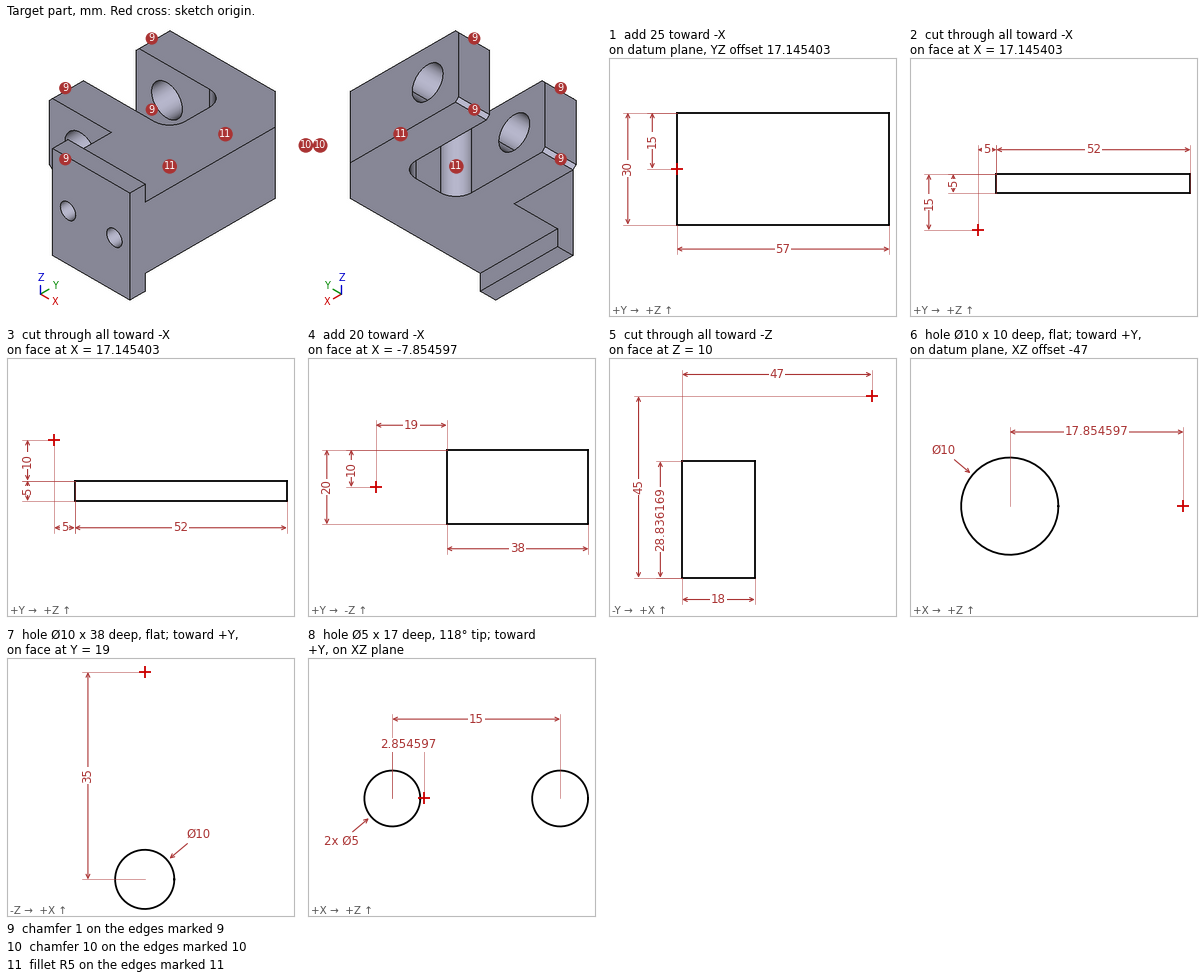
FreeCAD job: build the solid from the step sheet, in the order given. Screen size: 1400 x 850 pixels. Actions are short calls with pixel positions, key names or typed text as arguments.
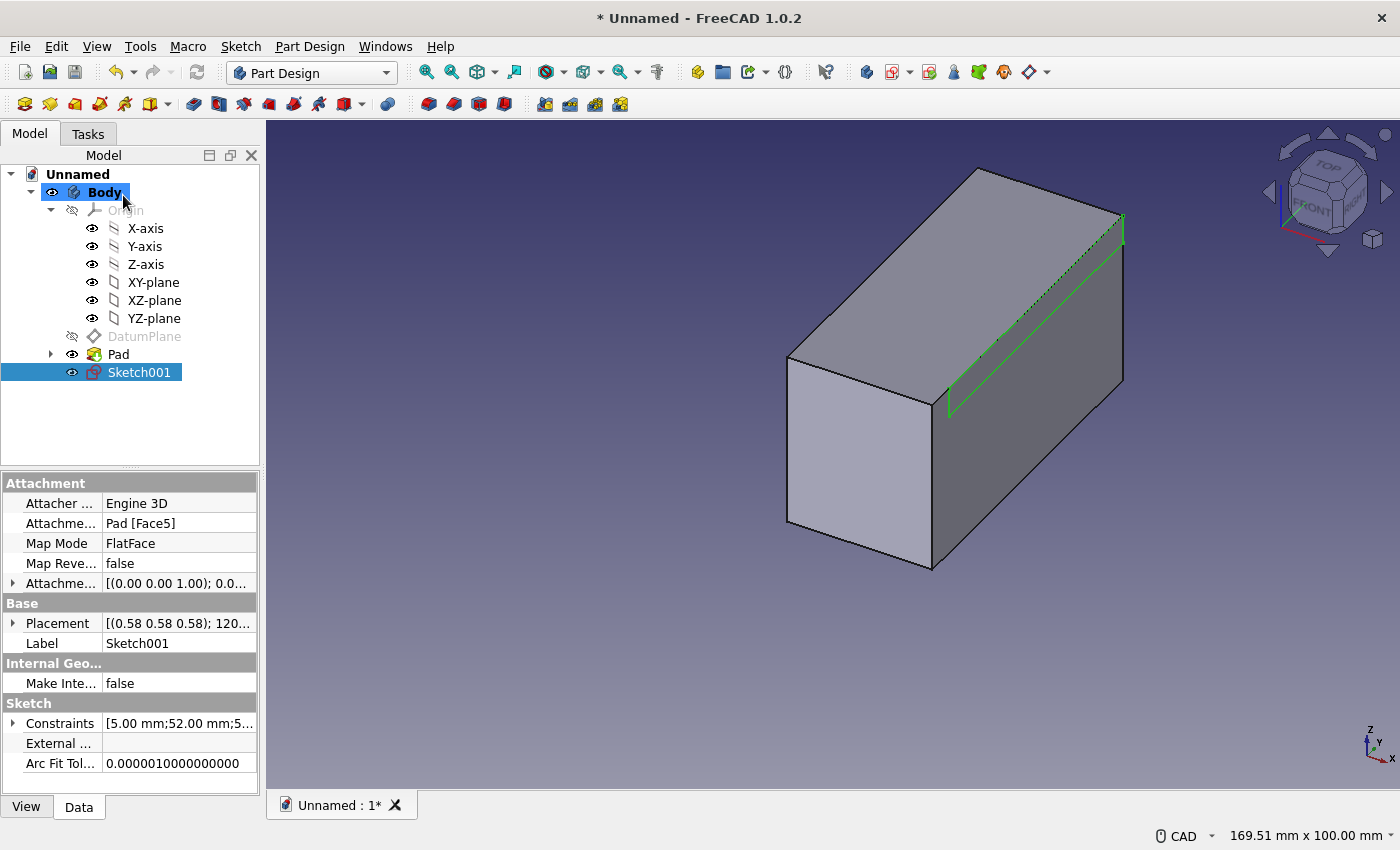
click(194, 104)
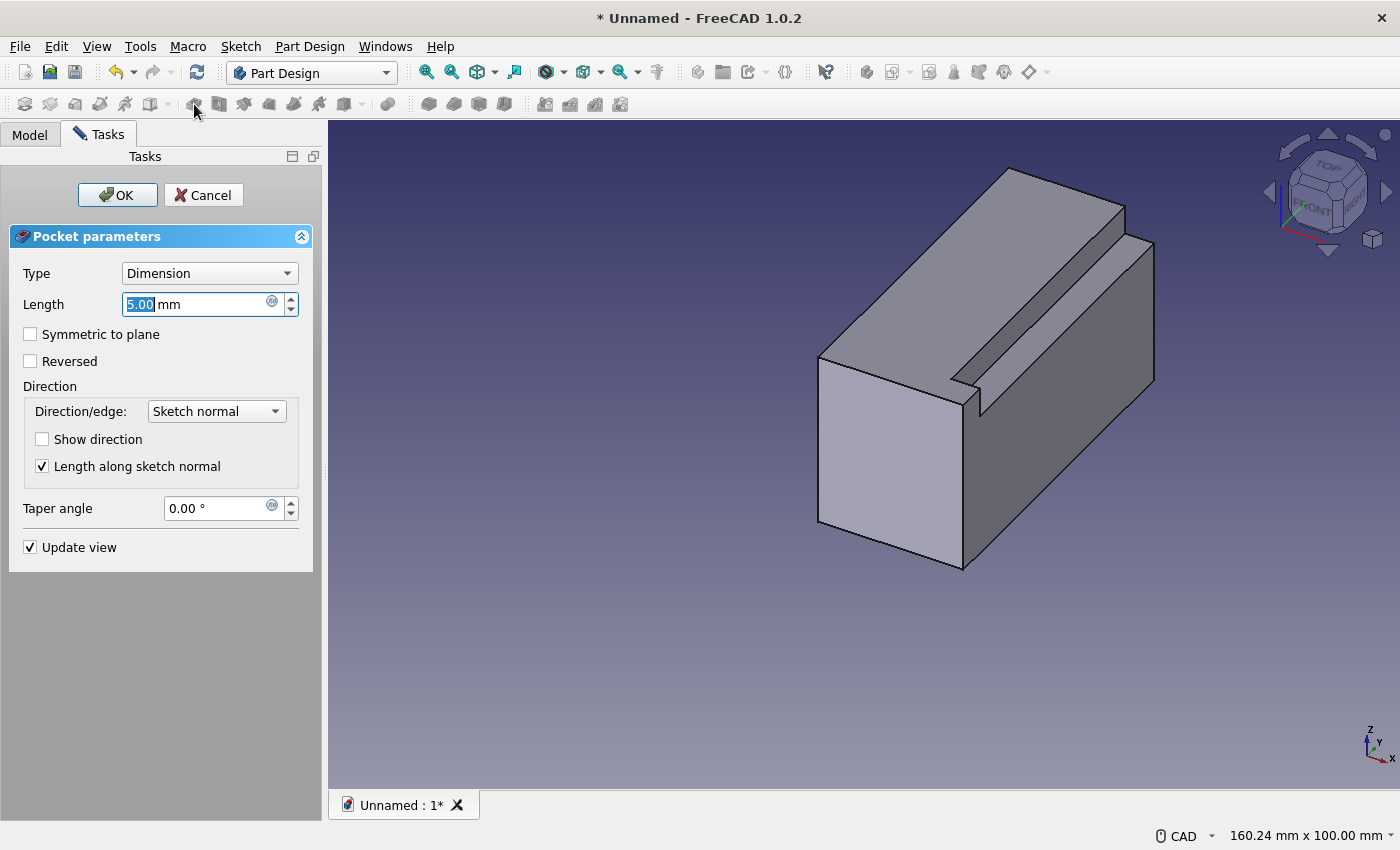
click(210, 274)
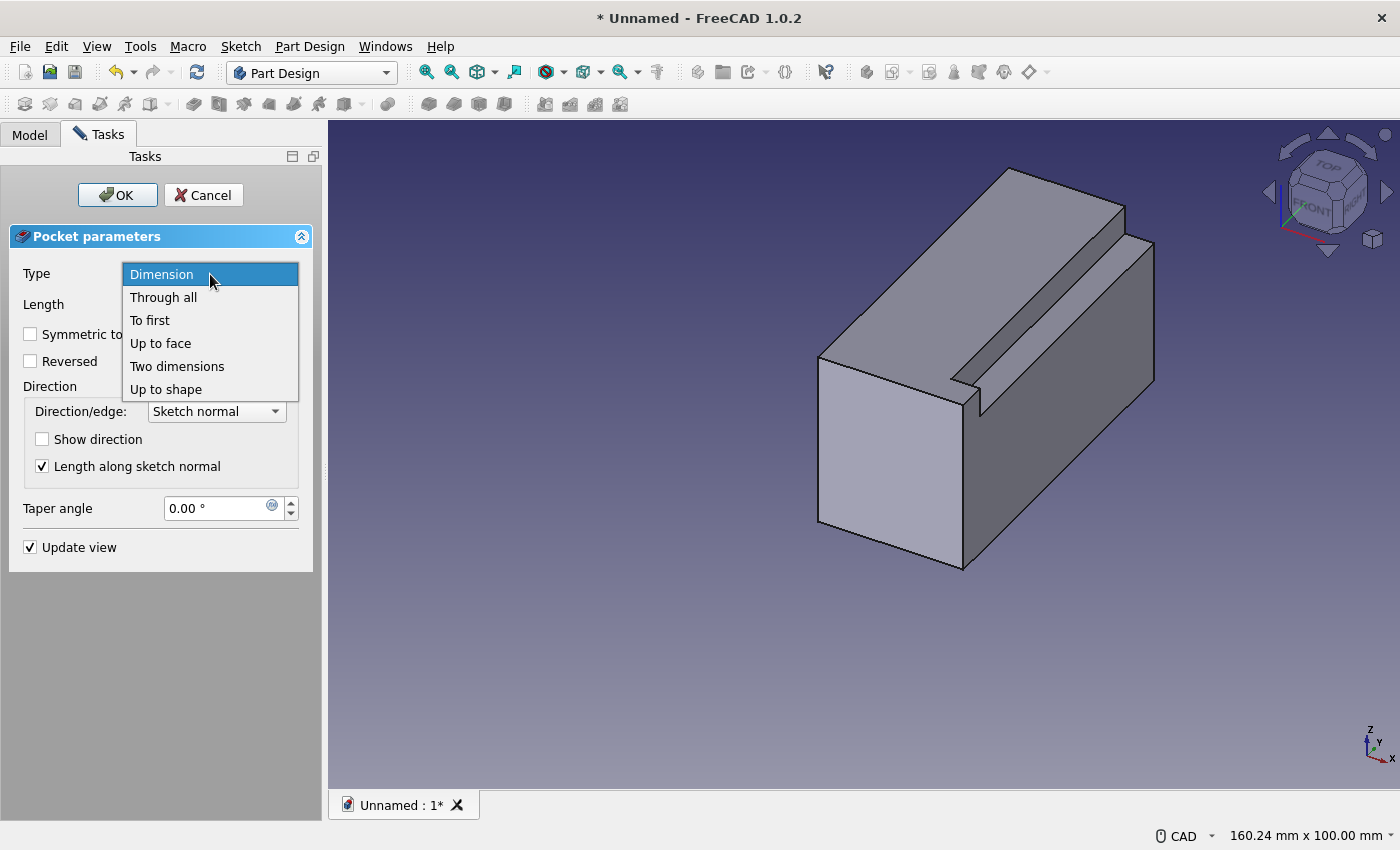
click(208, 298)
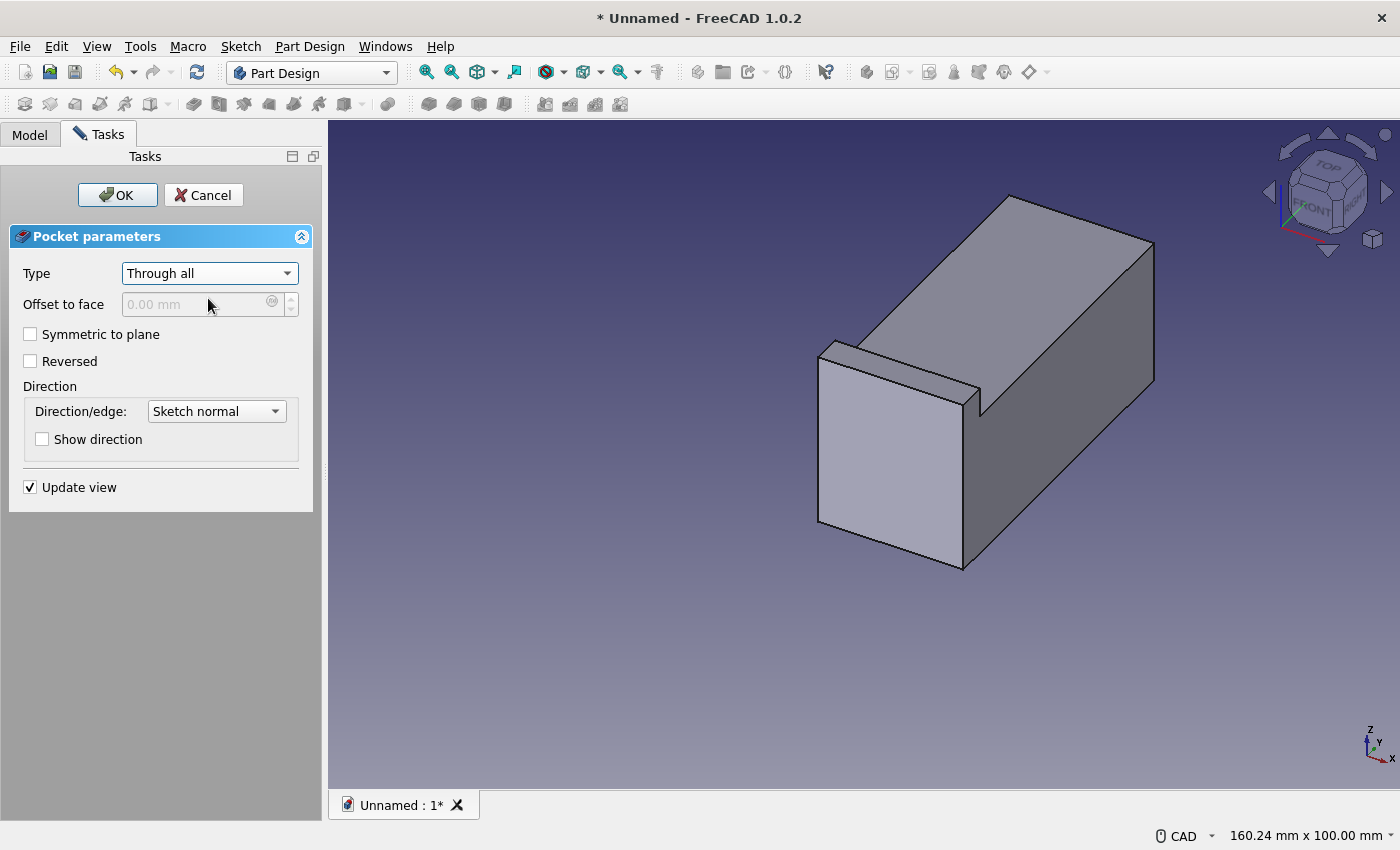
click(118, 195)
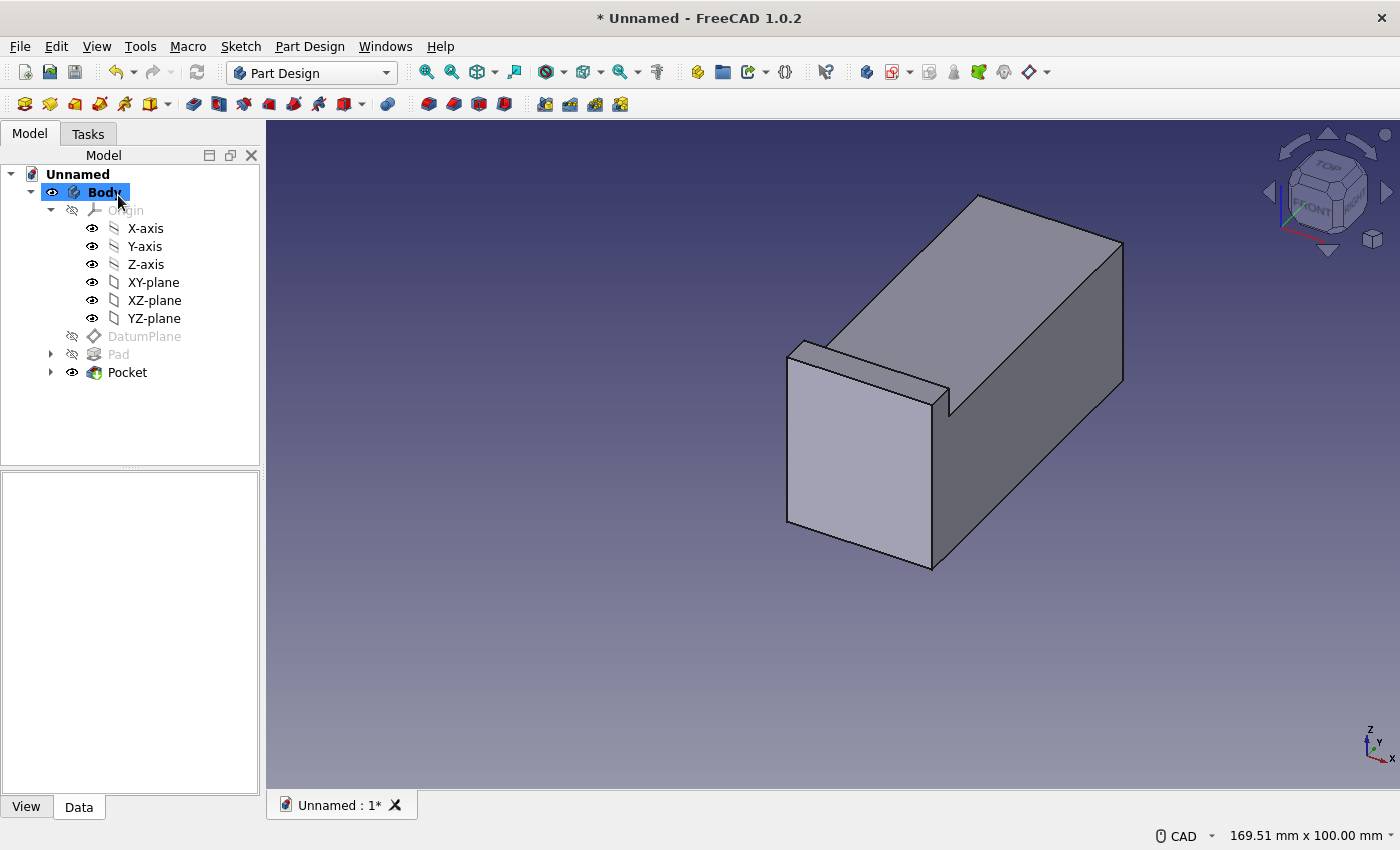
click(1082, 361)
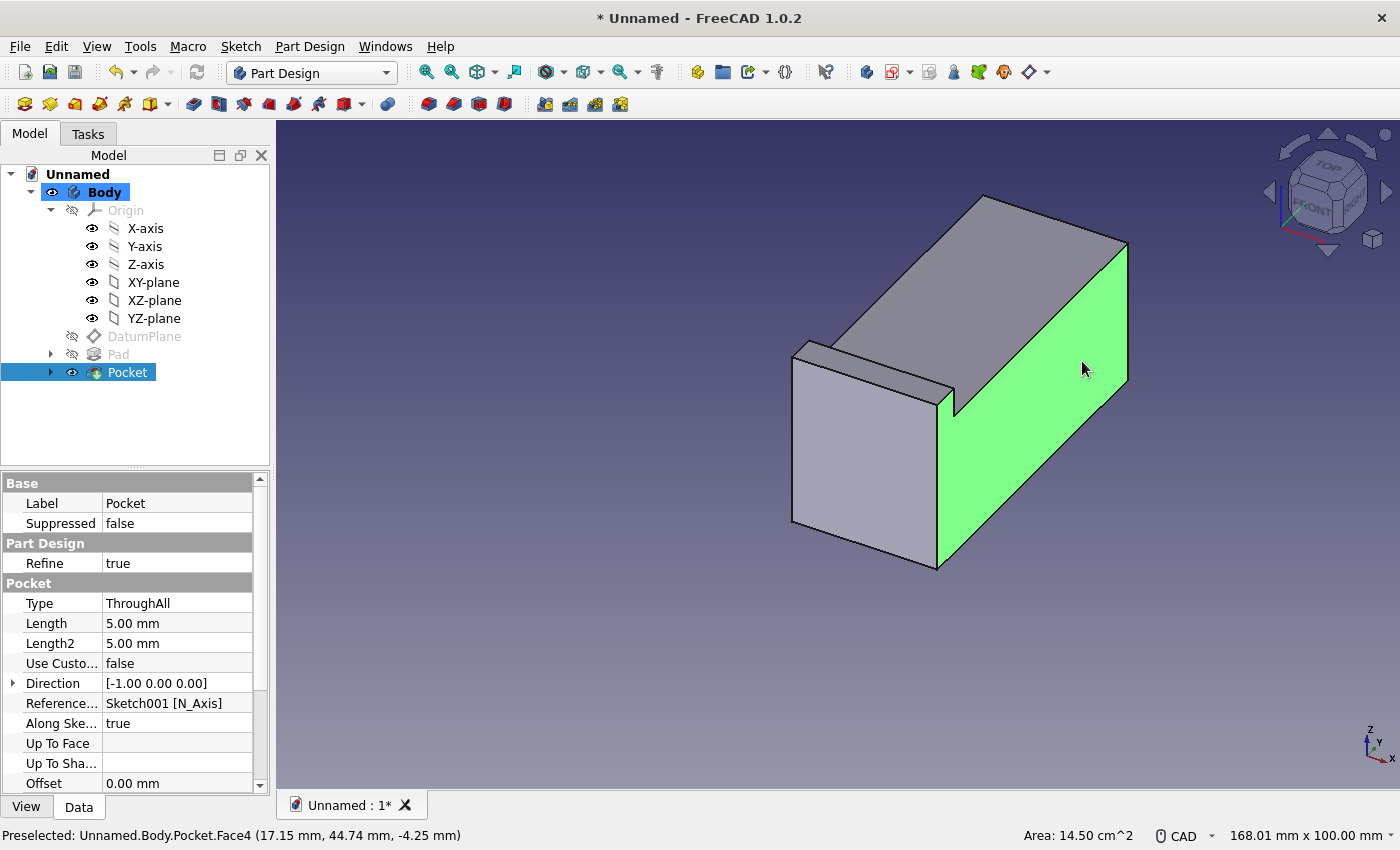
click(892, 72)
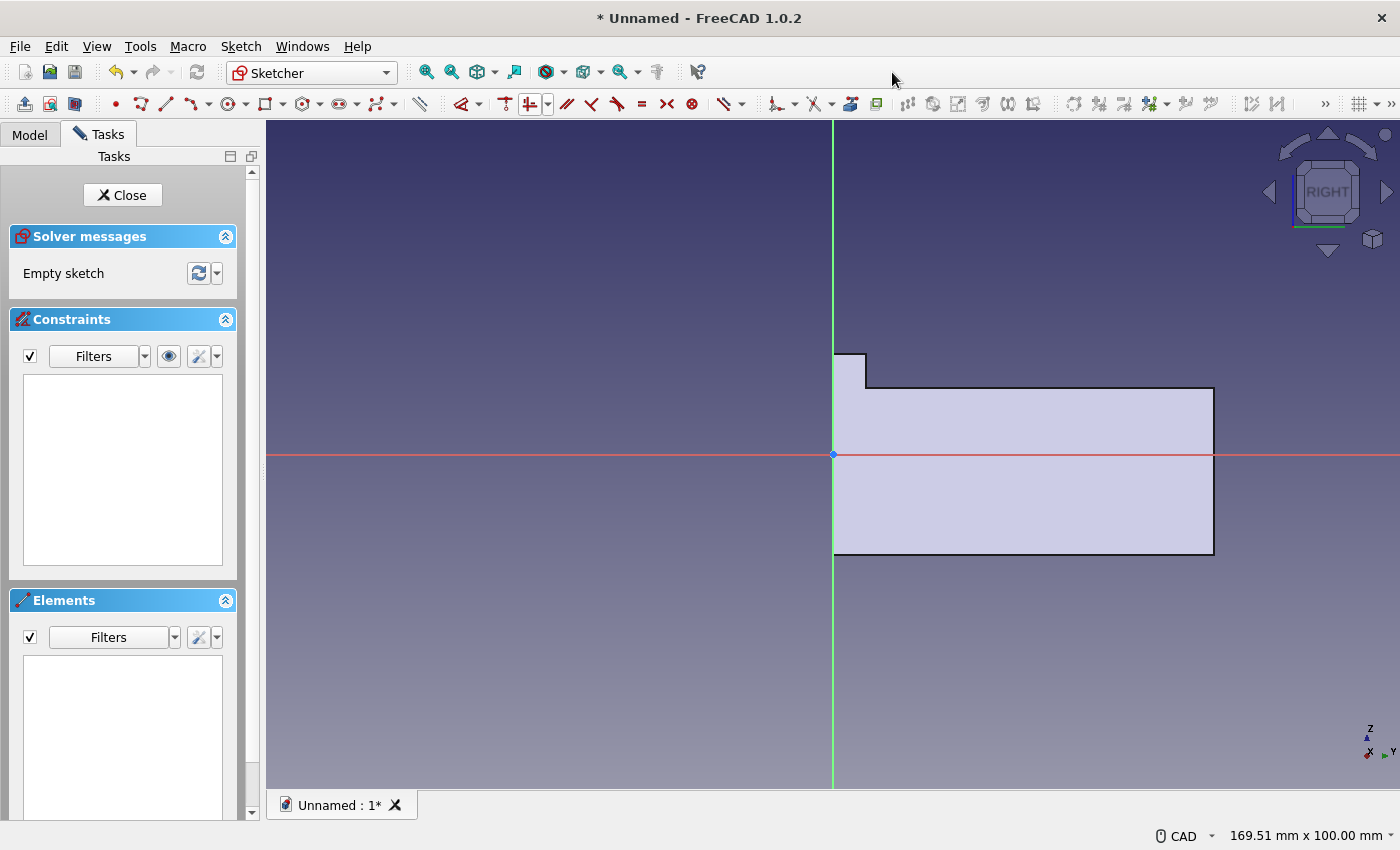
scroll(1235, 566, up, 3)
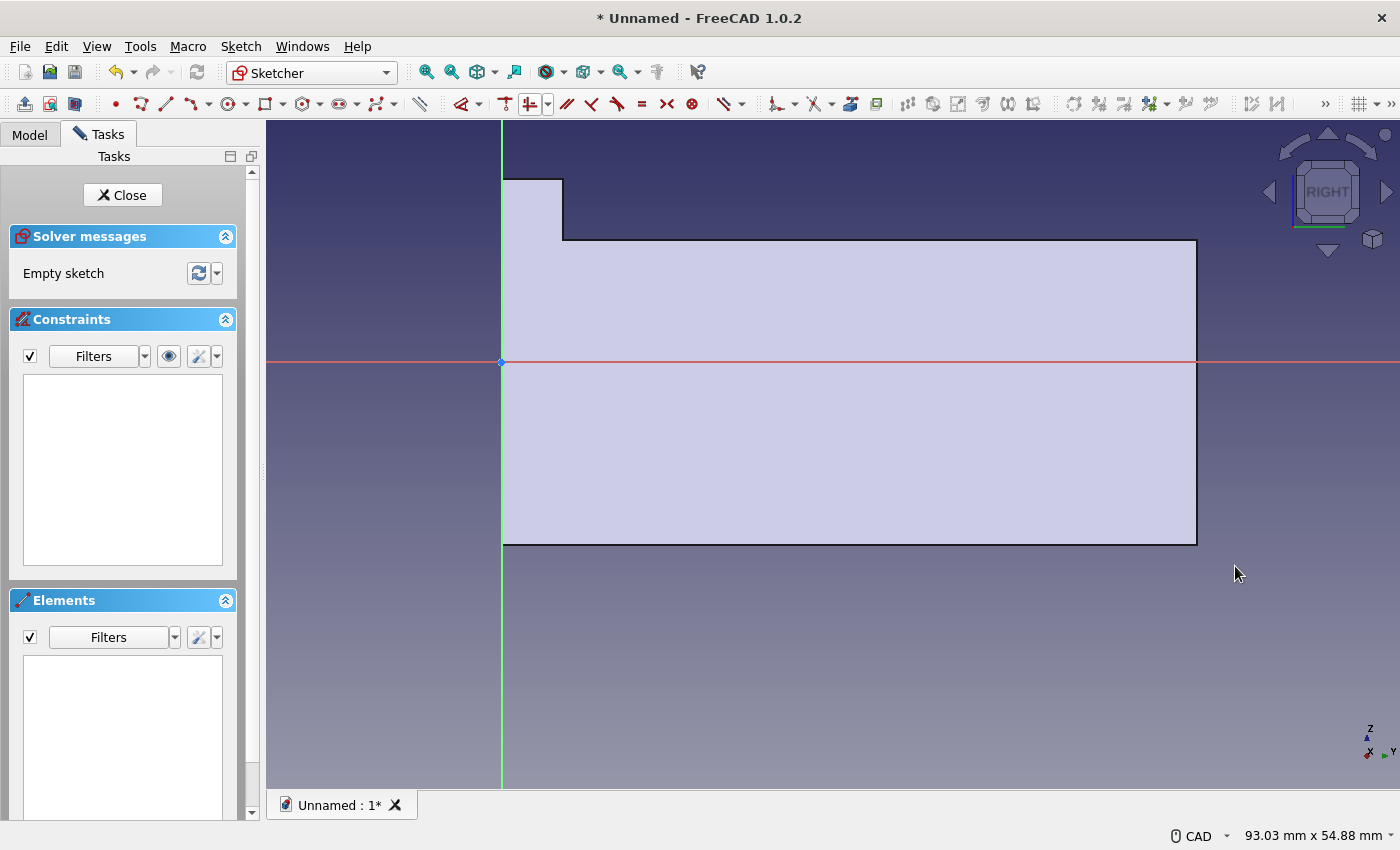
click(264, 104)